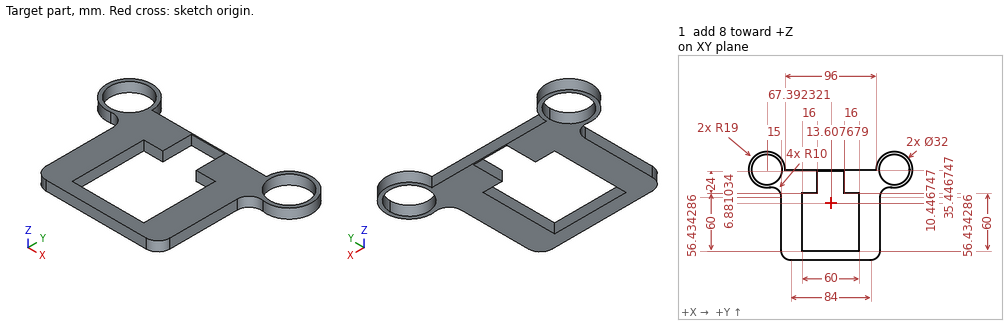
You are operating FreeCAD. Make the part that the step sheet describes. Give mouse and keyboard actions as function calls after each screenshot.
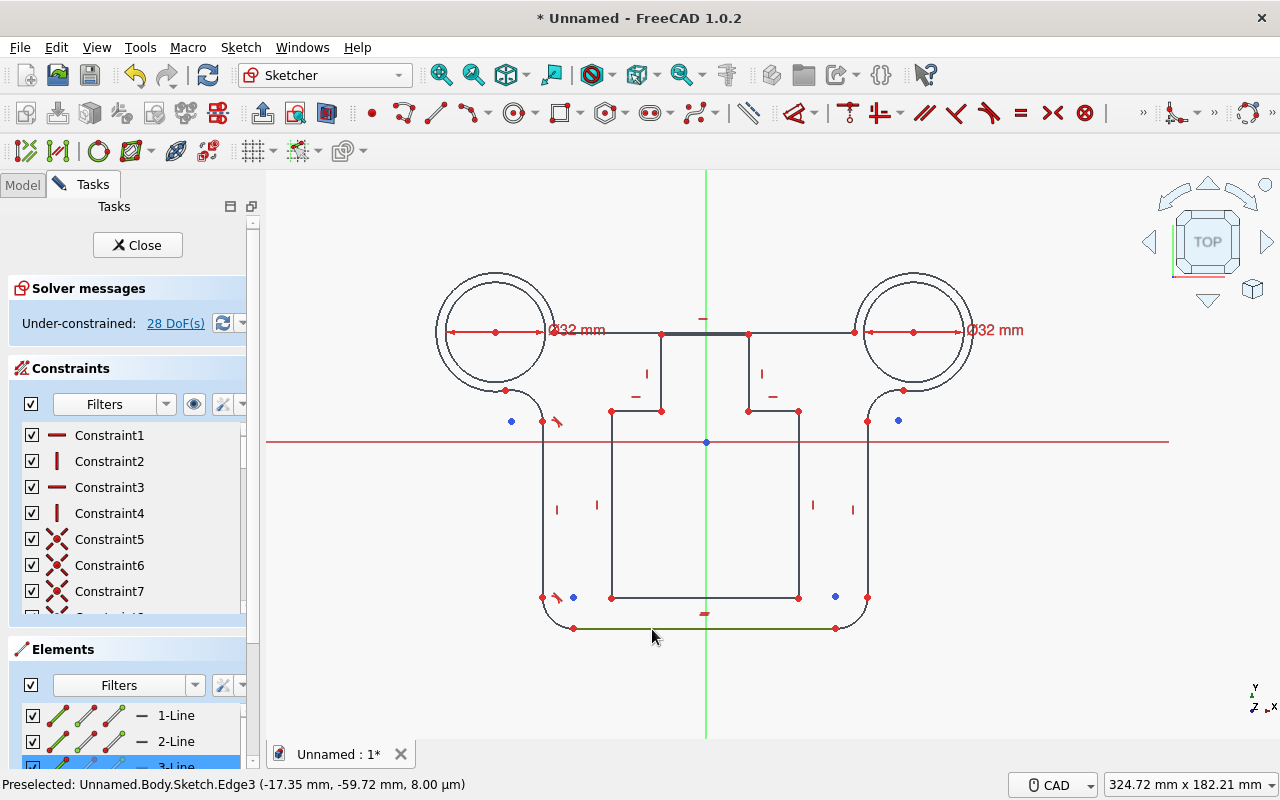
click(546, 612)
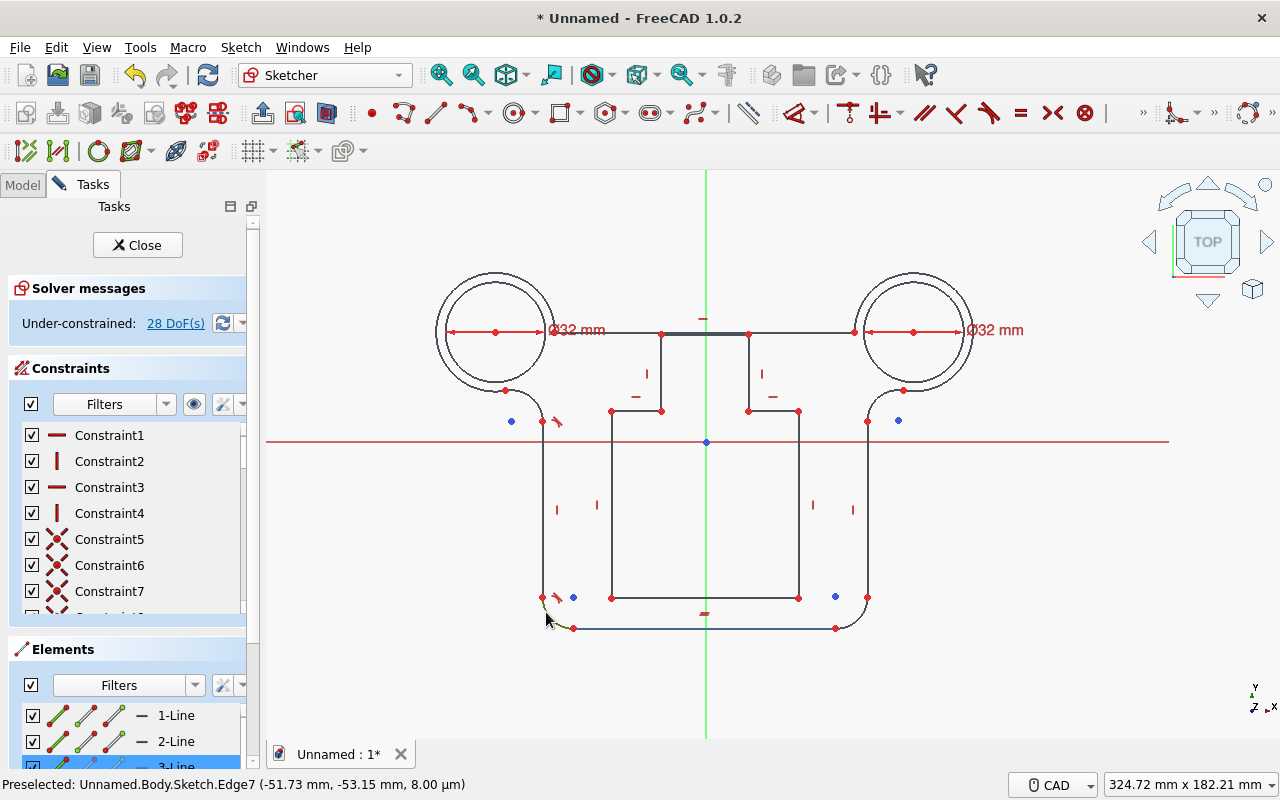
click(990, 114)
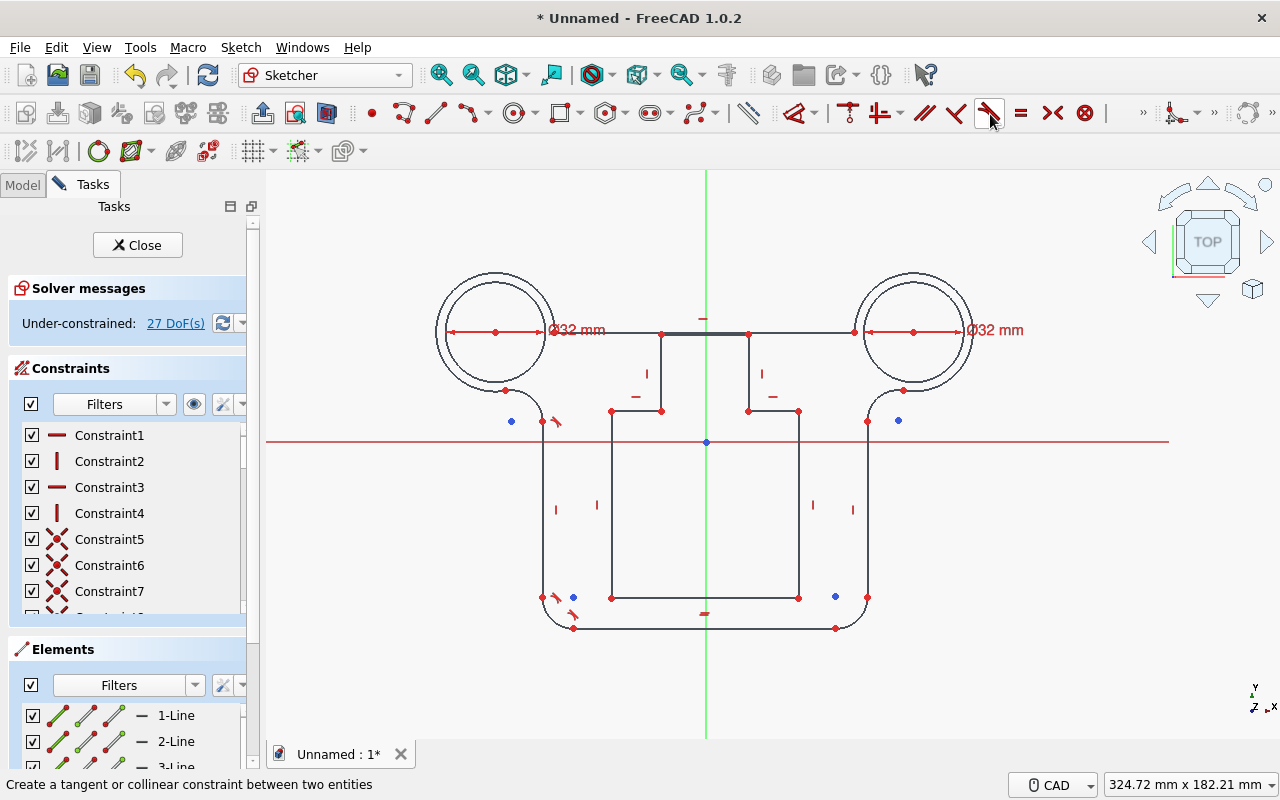
click(652, 629)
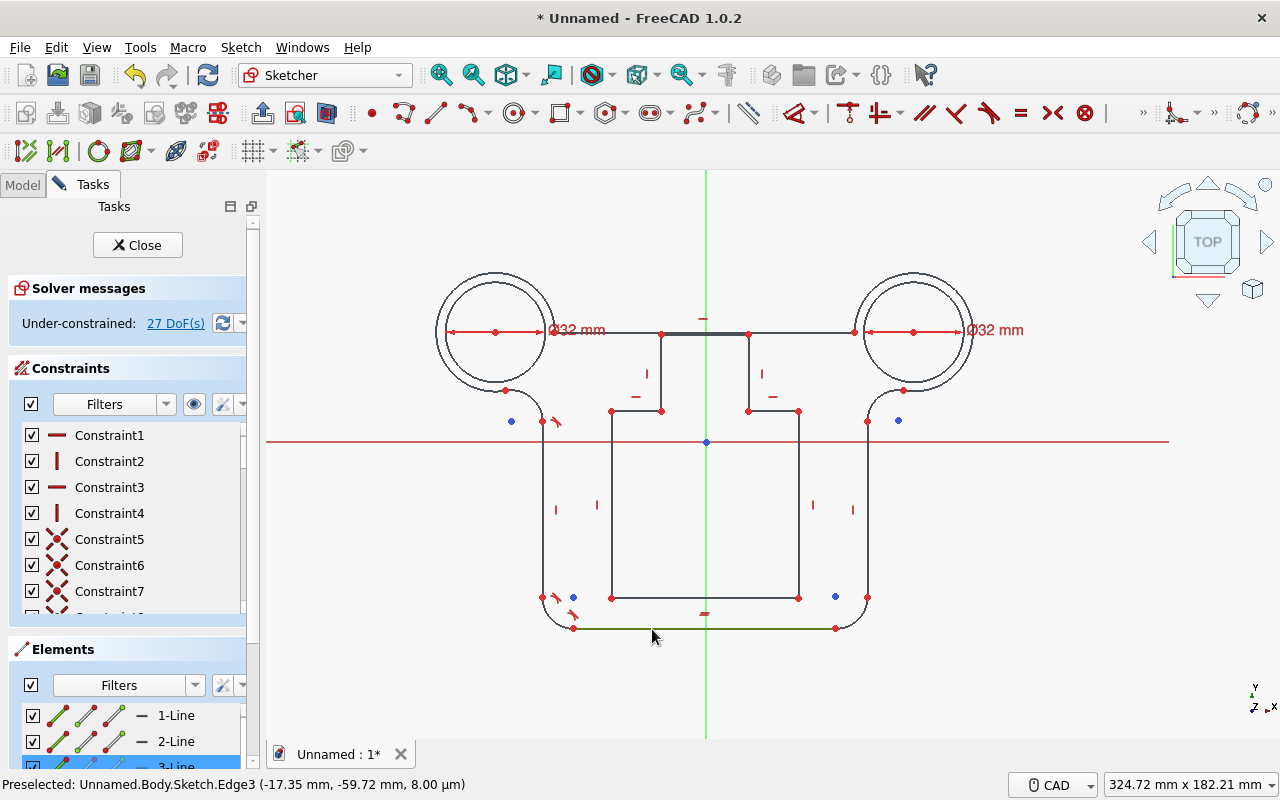
click(850, 625)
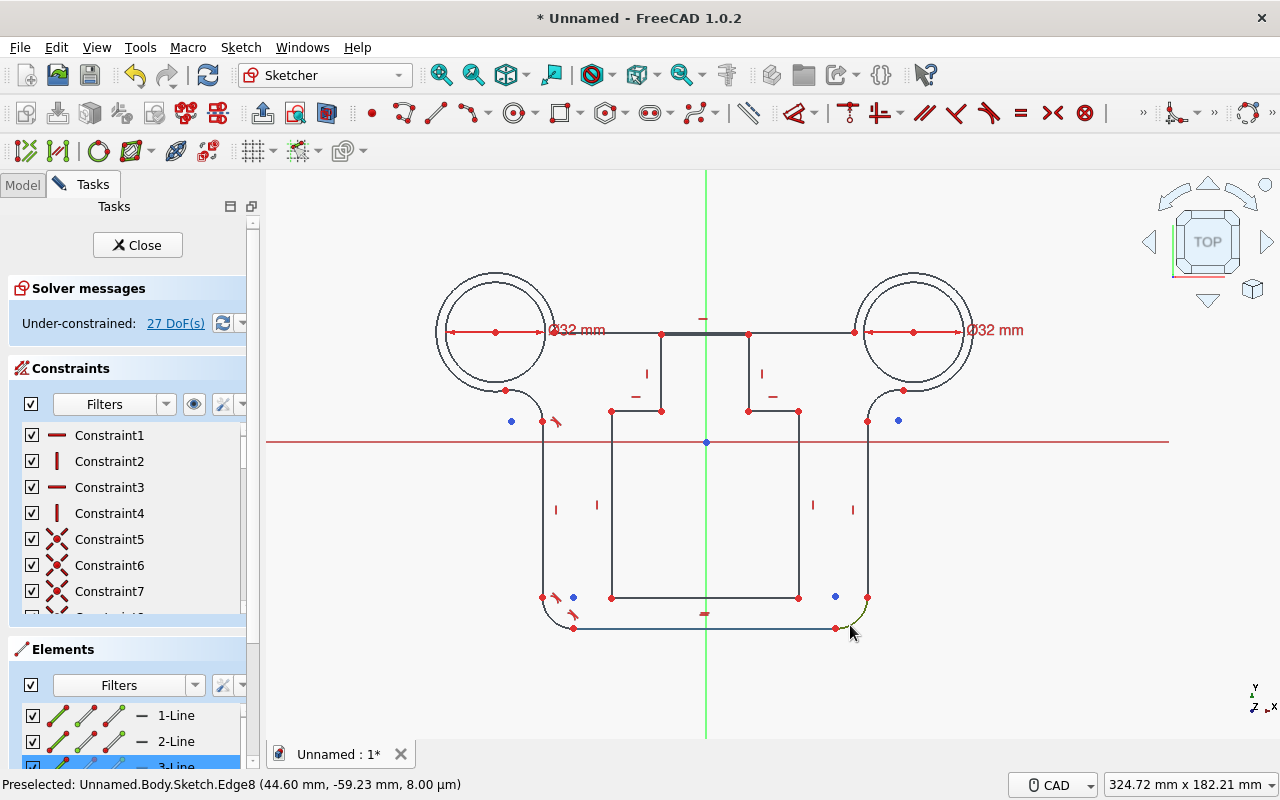
click(990, 114)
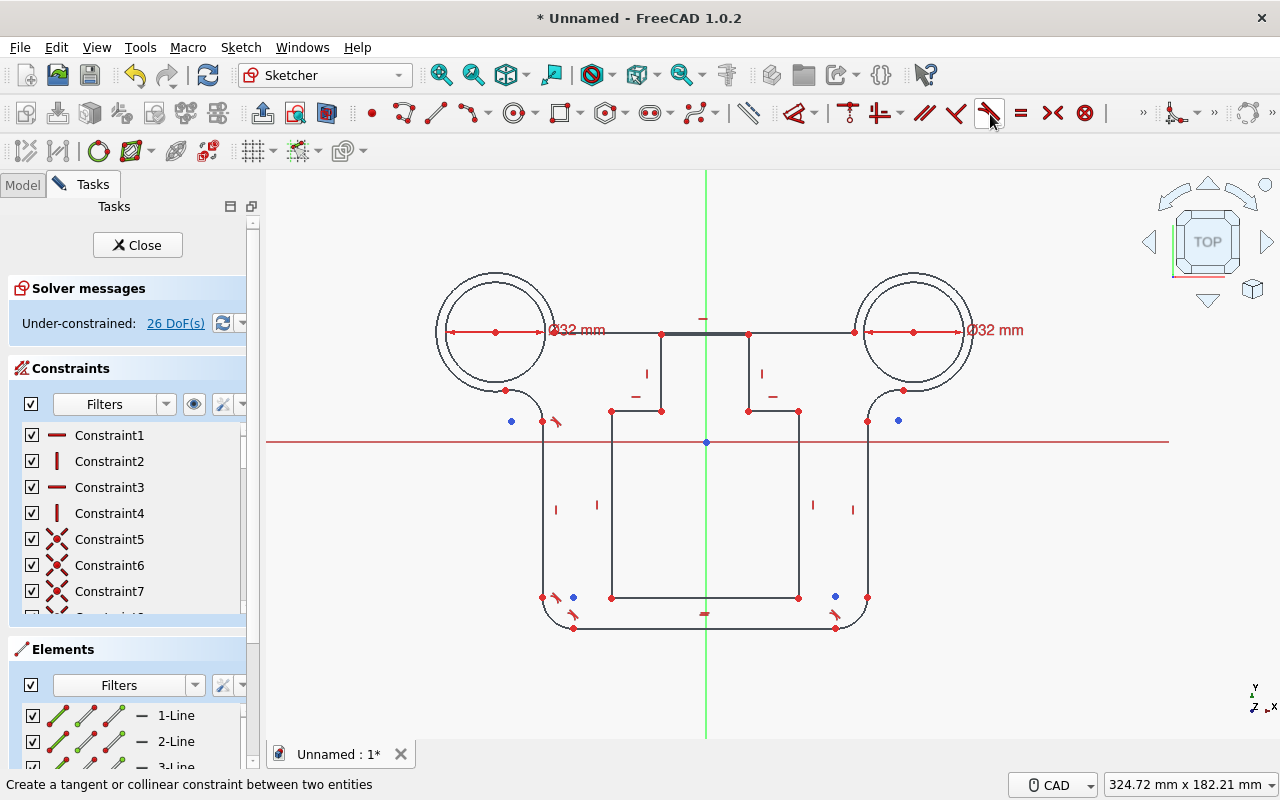
click(868, 545)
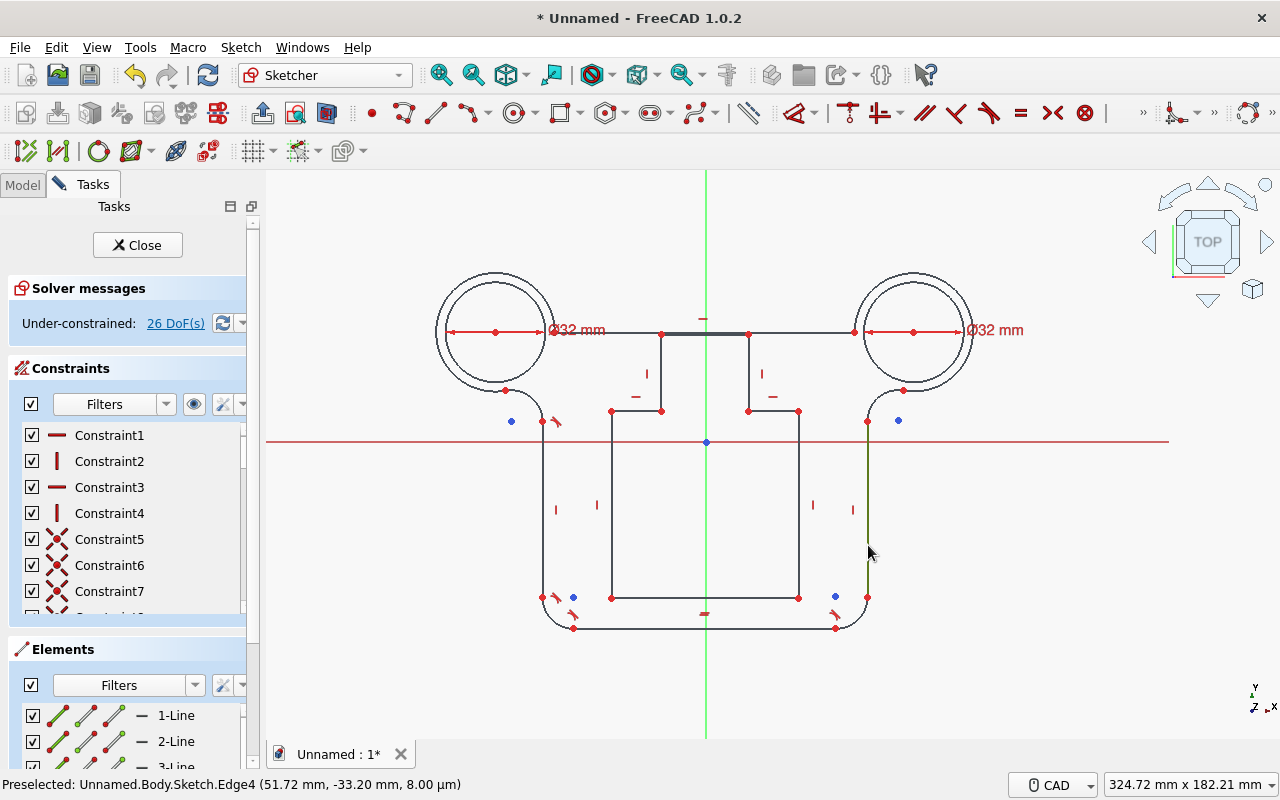
click(850, 626)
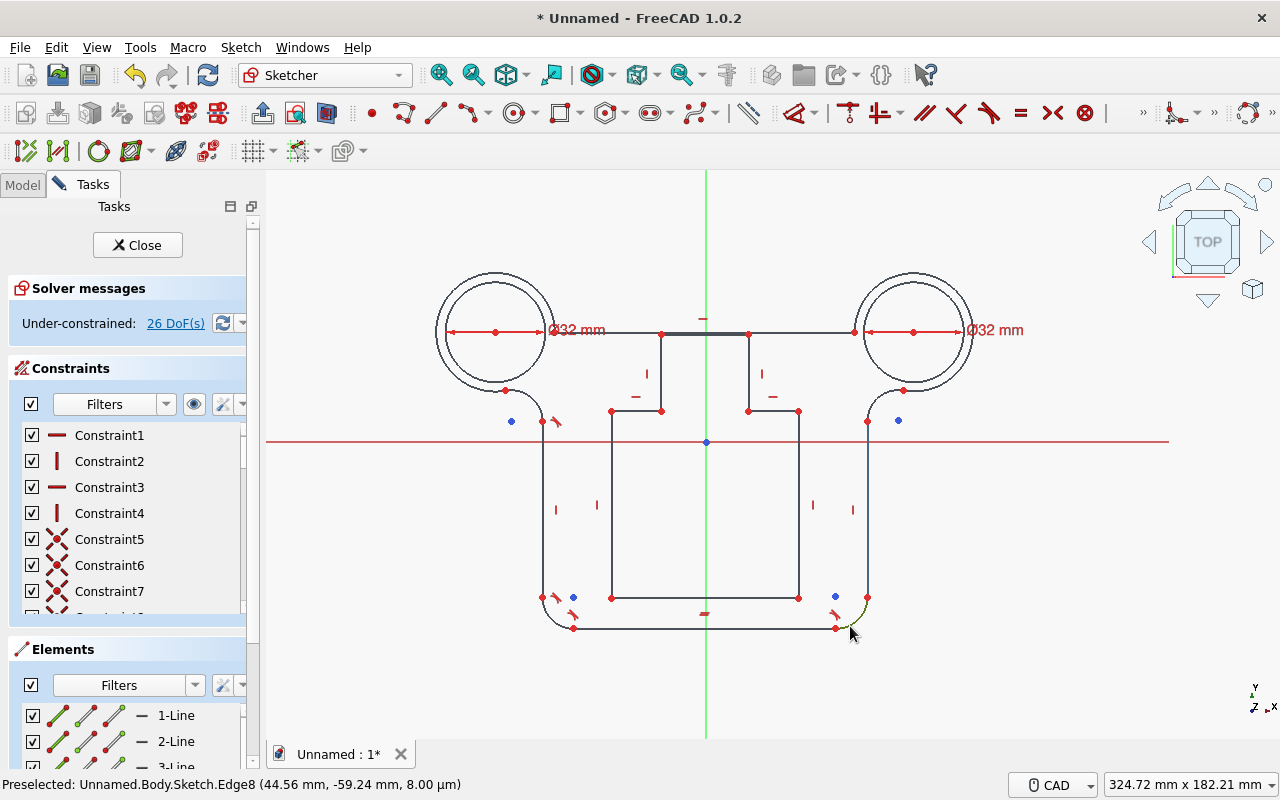
click(990, 114)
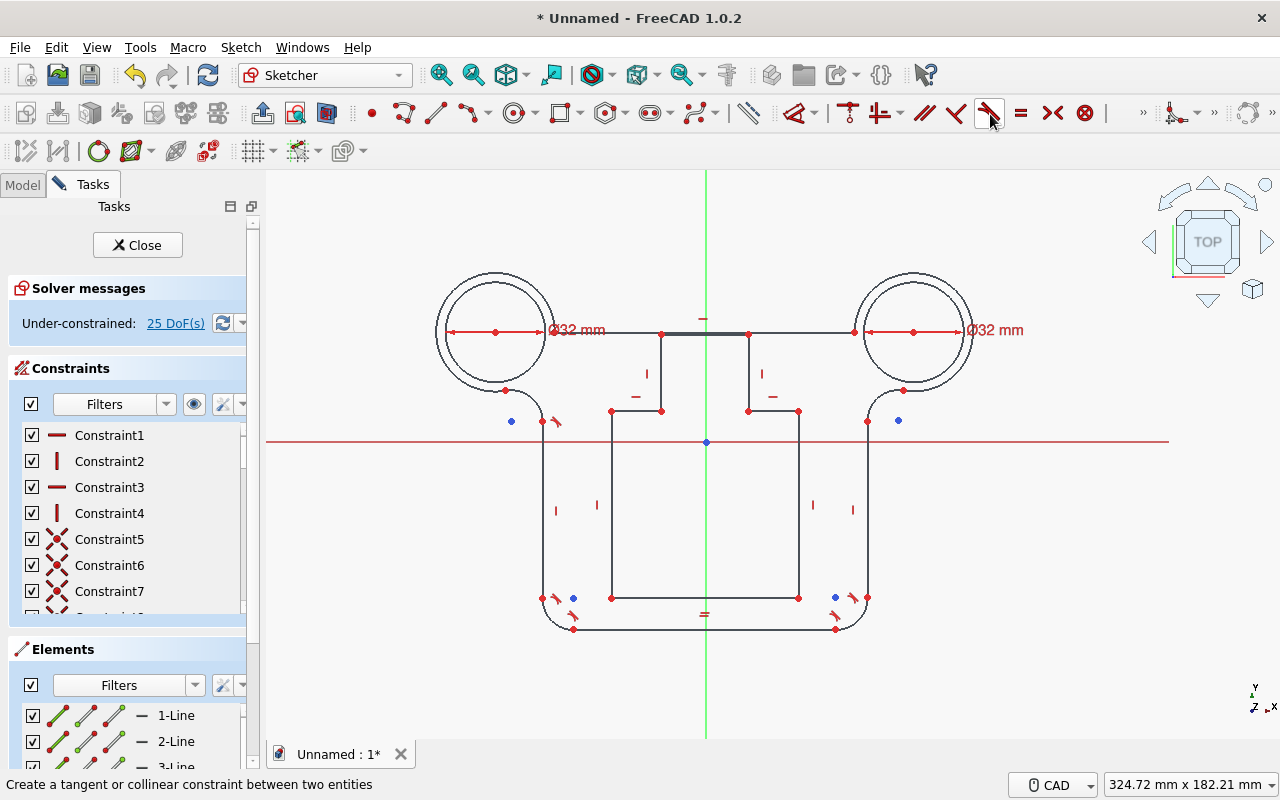
click(868, 545)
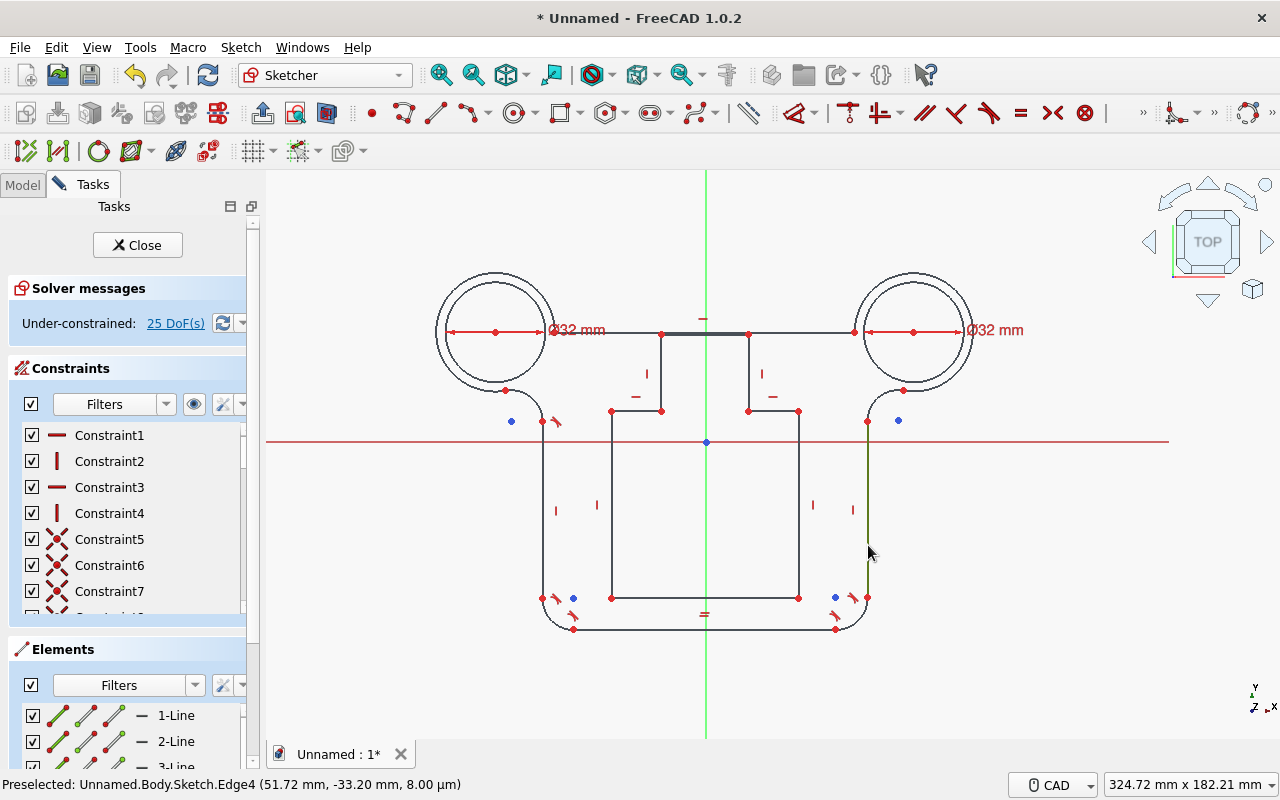
click(888, 392)